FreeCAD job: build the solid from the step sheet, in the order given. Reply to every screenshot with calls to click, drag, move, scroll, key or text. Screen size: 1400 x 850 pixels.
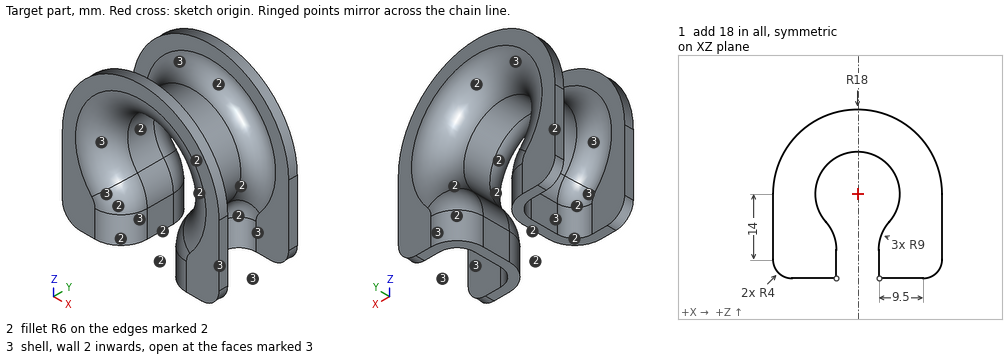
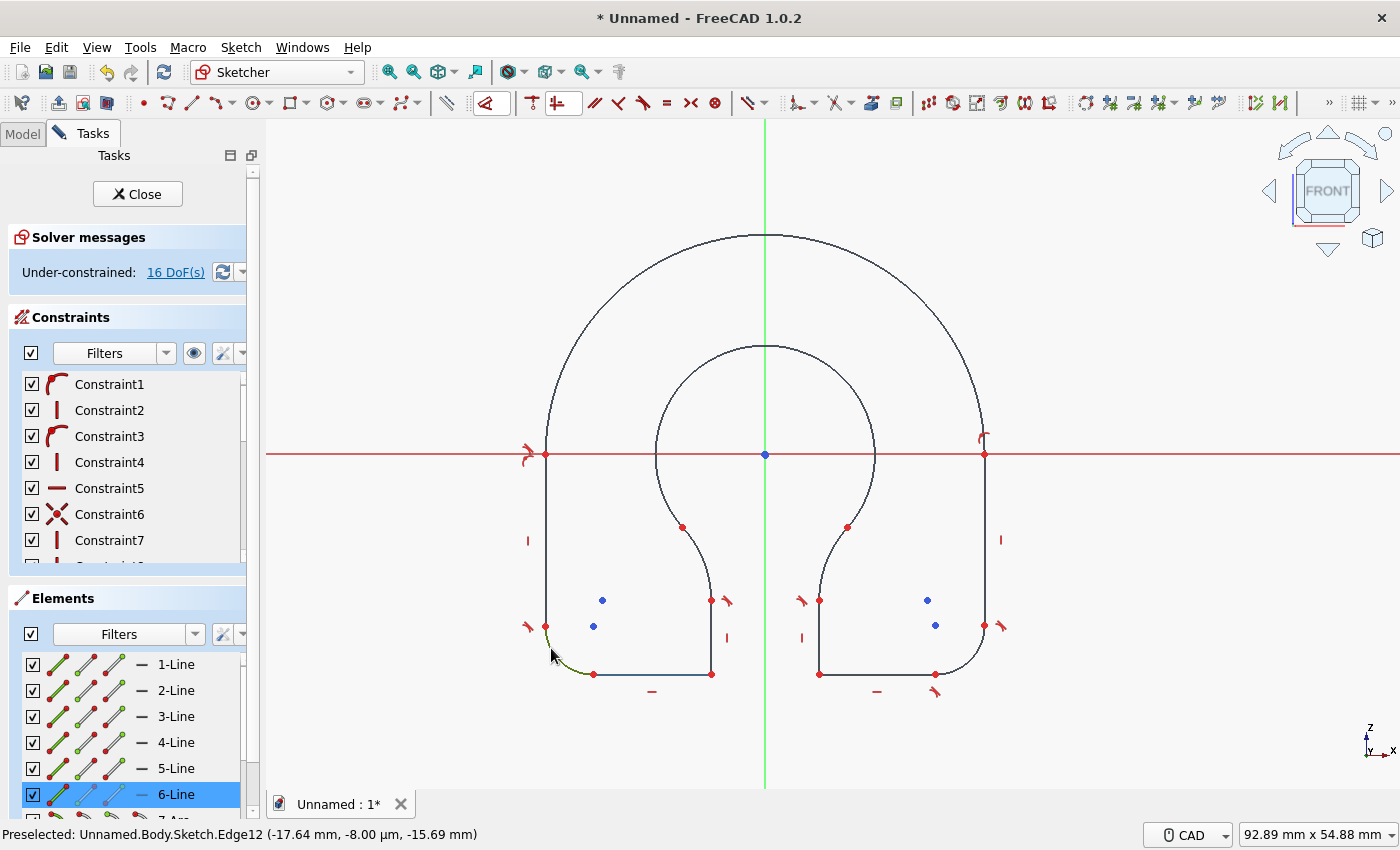
key(t)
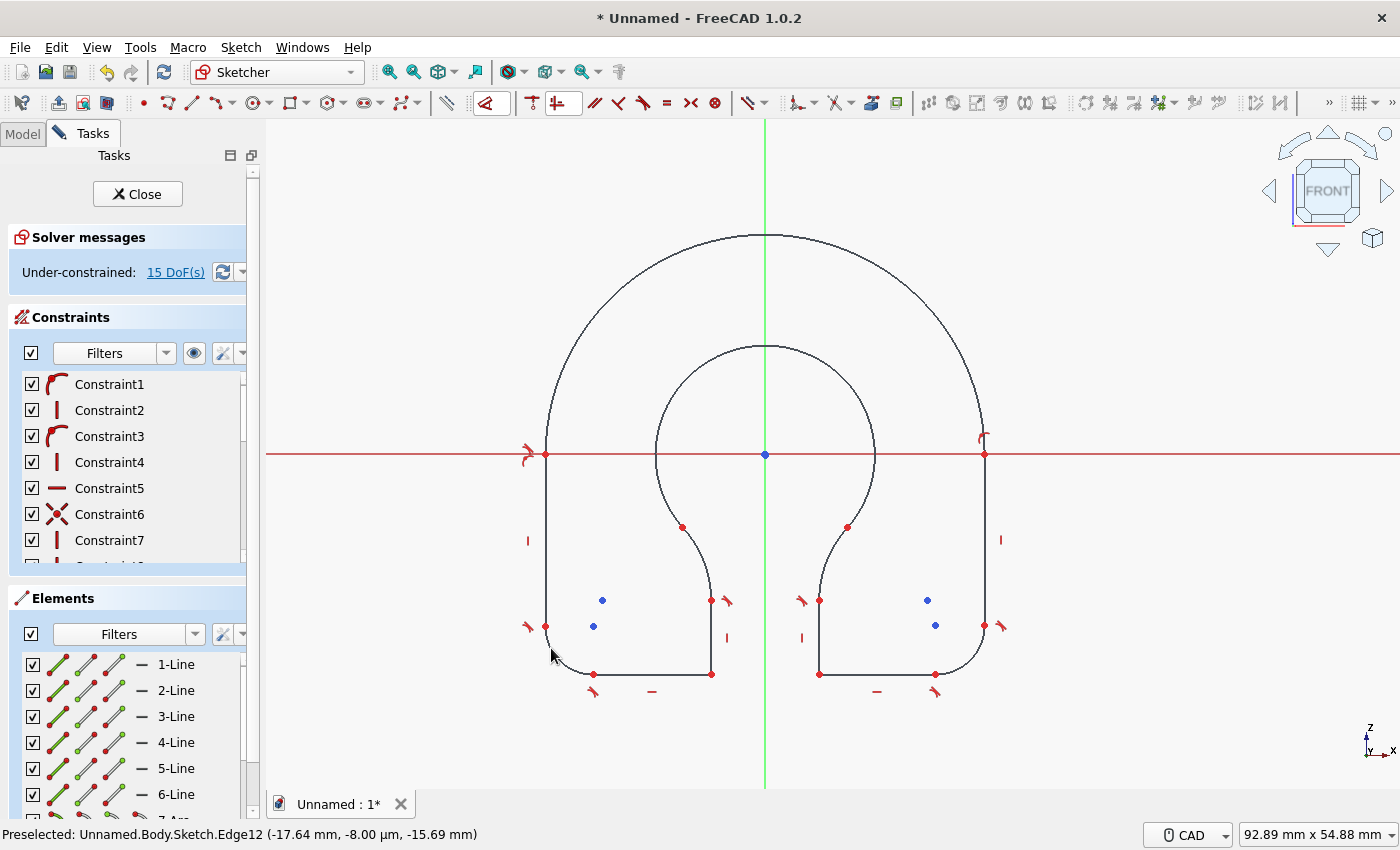
click(833, 547)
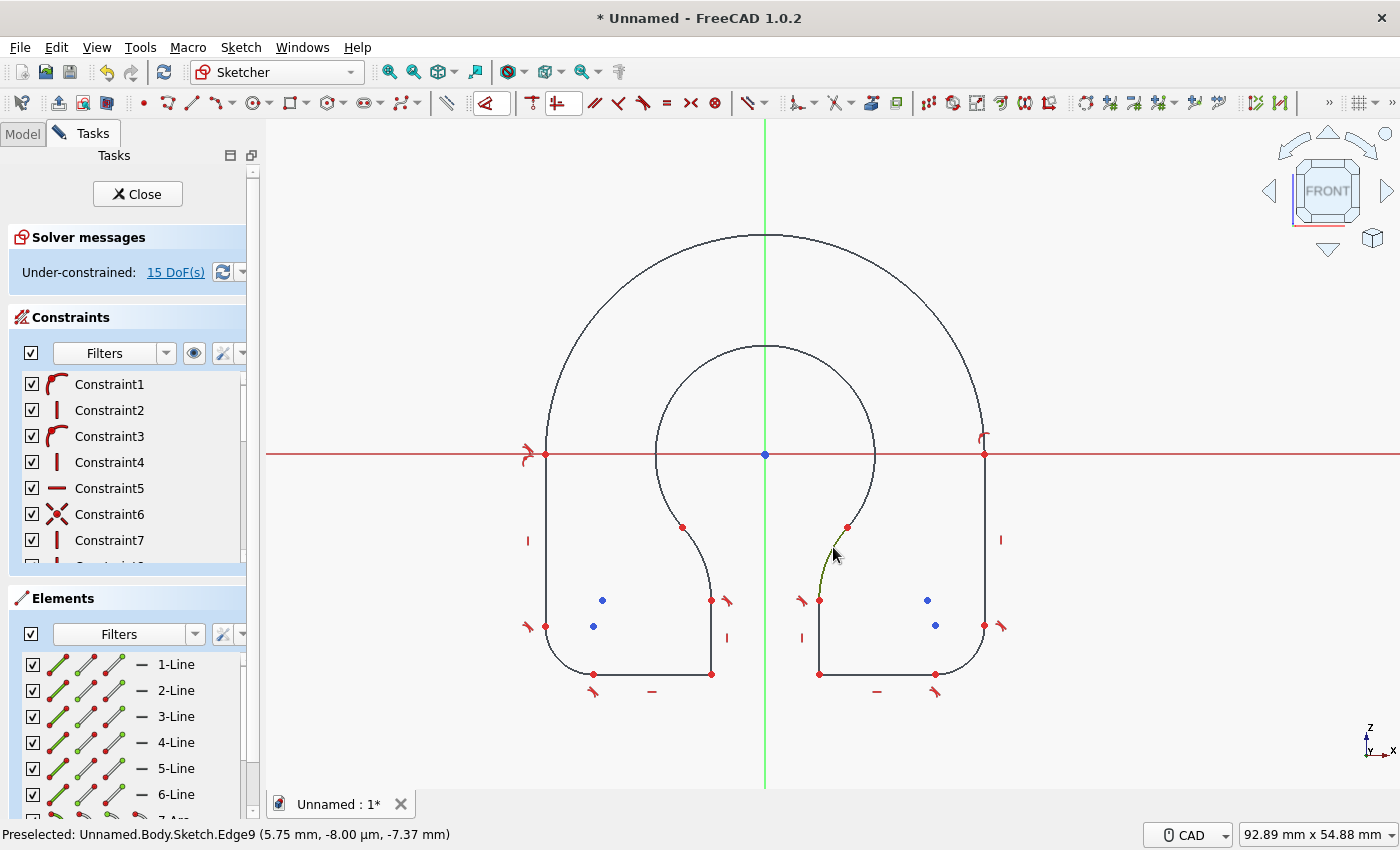
click(852, 389)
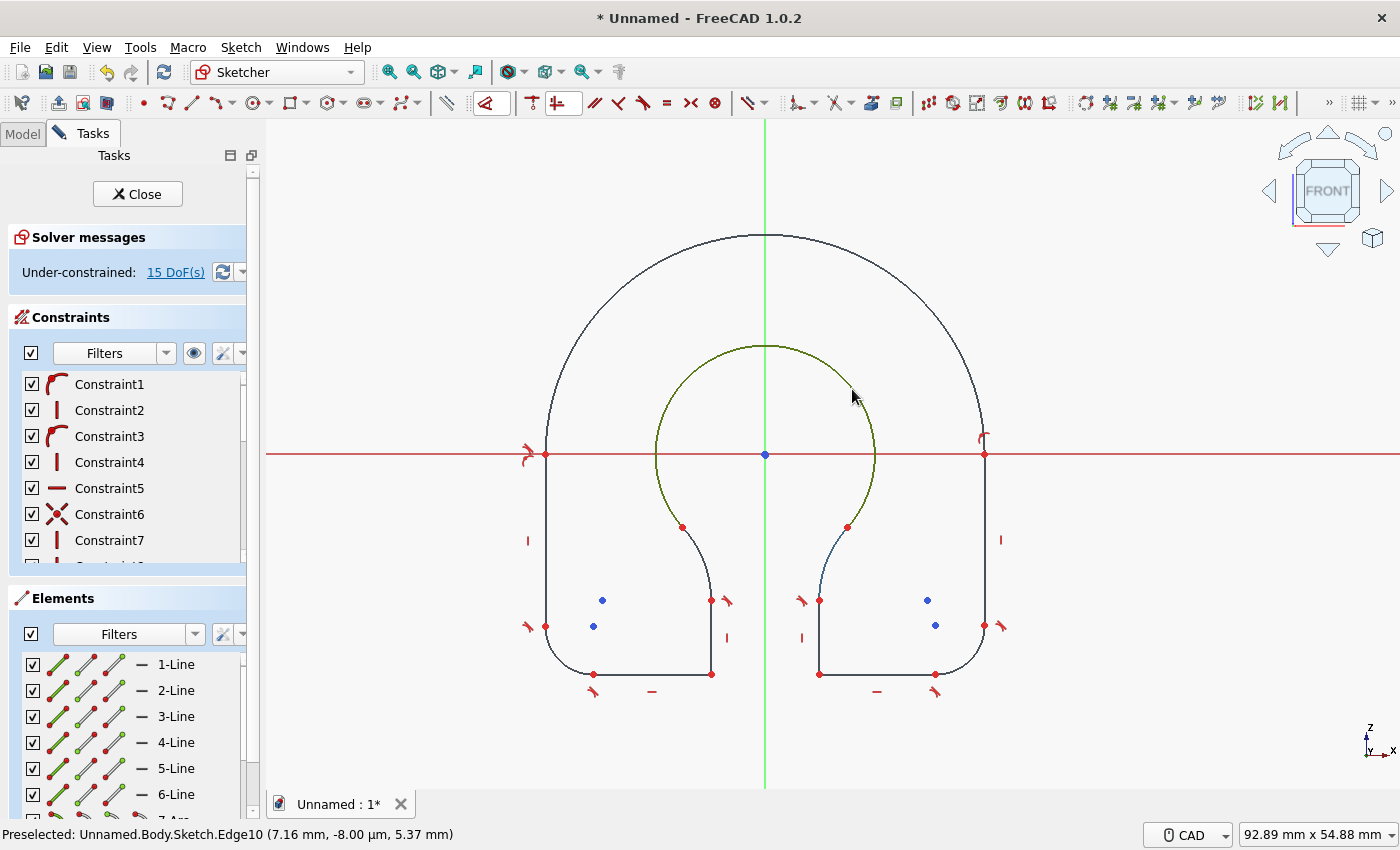
key(t)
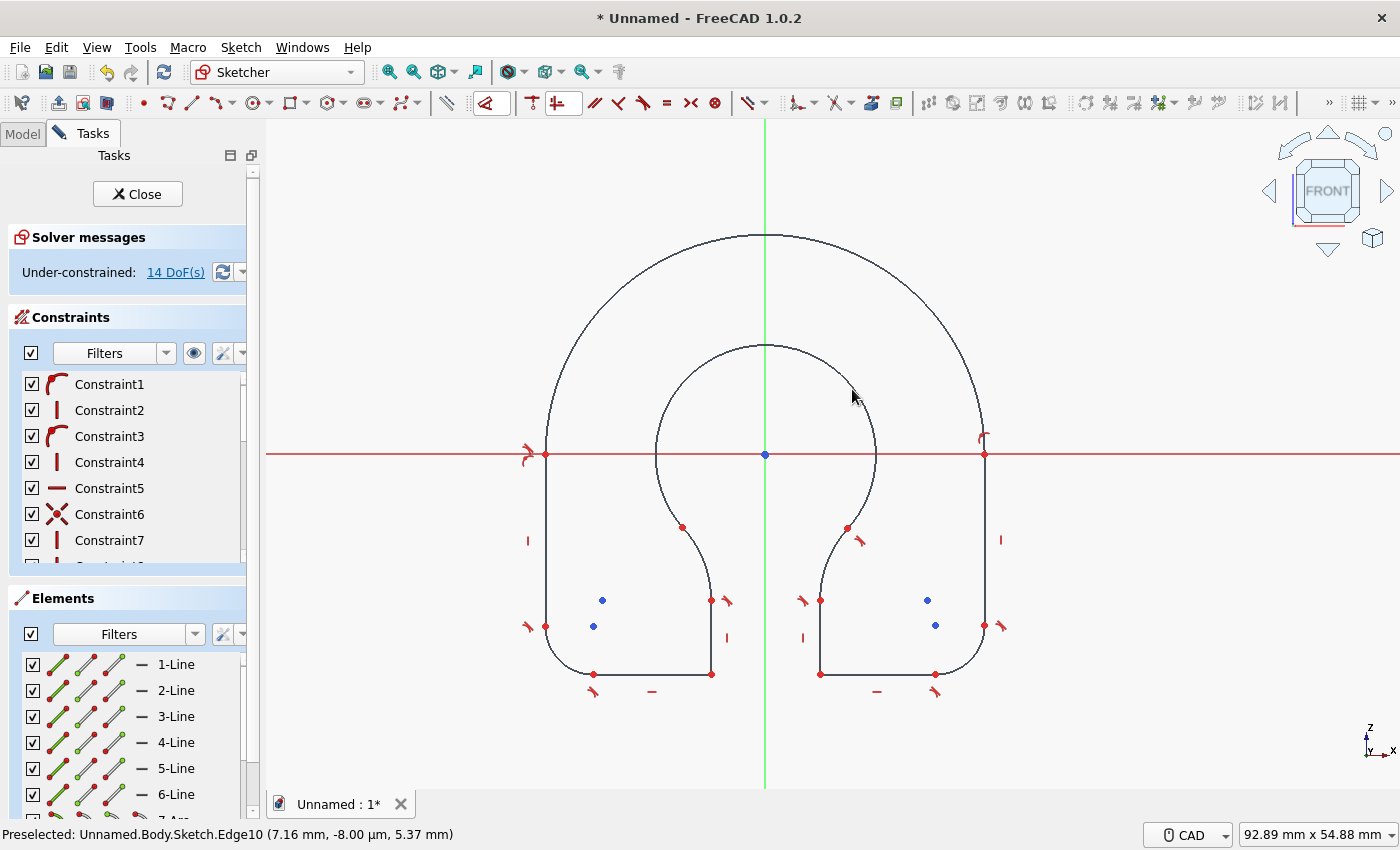
click(854, 389)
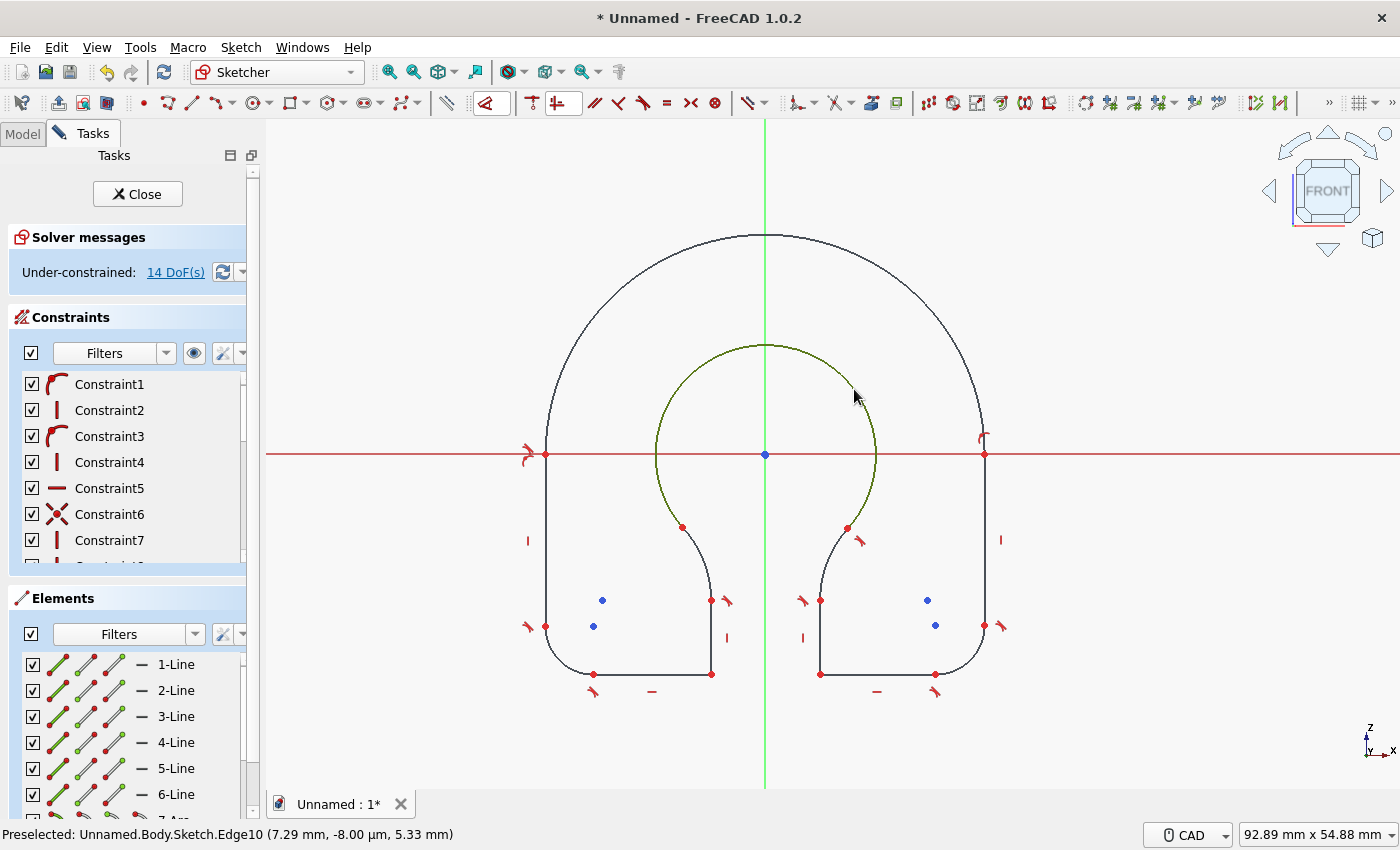
click(708, 577)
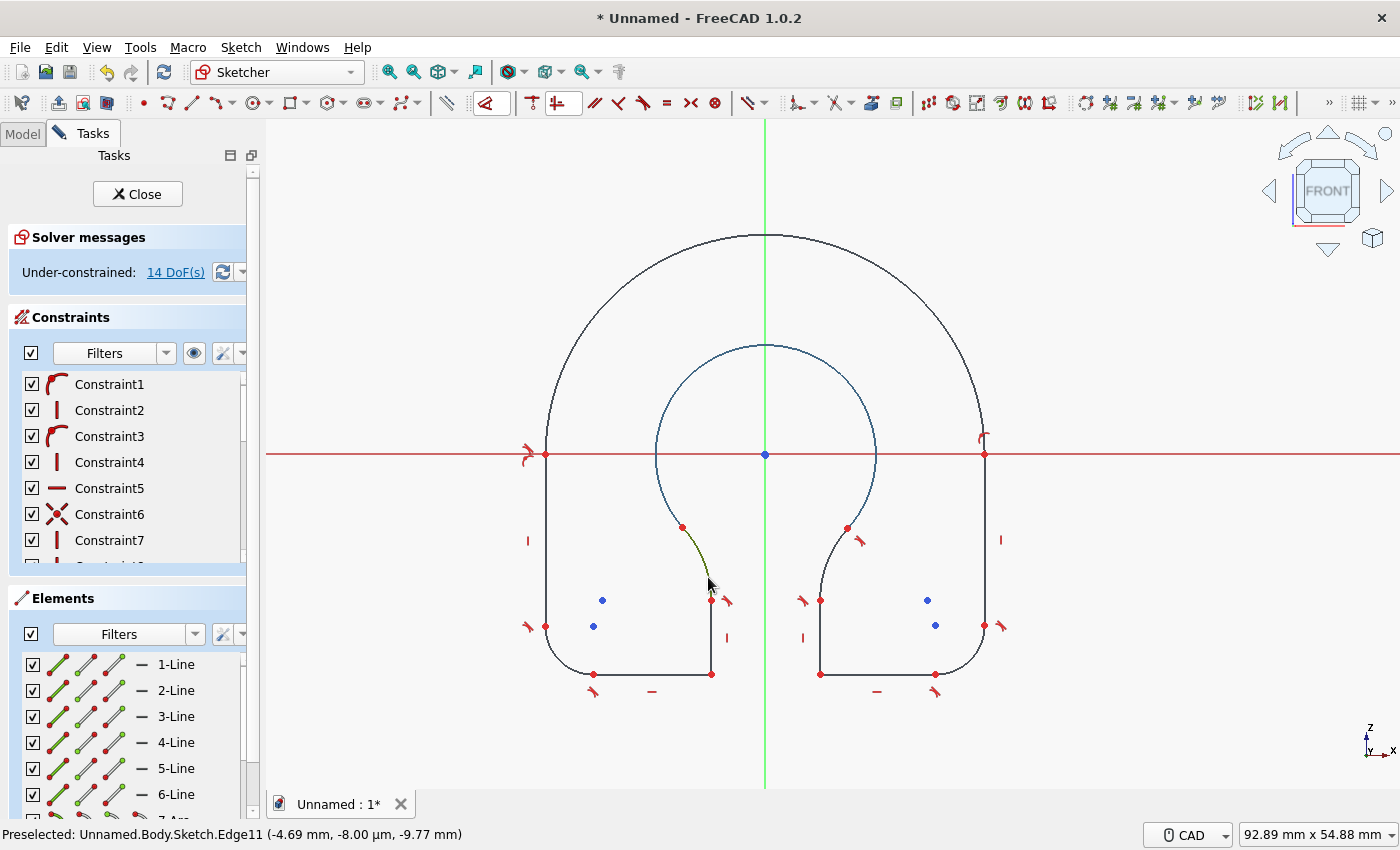
key(t)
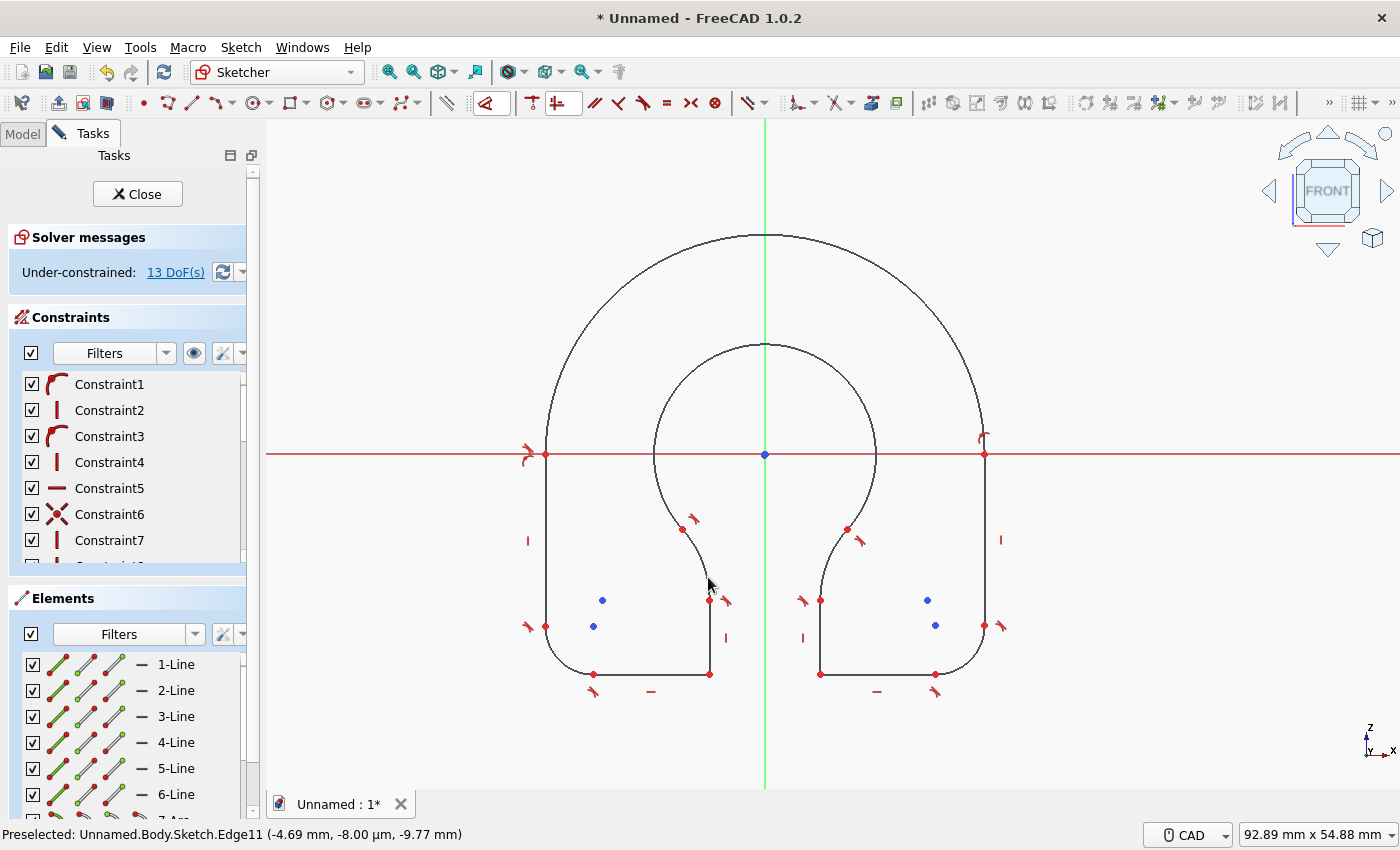
click(894, 277)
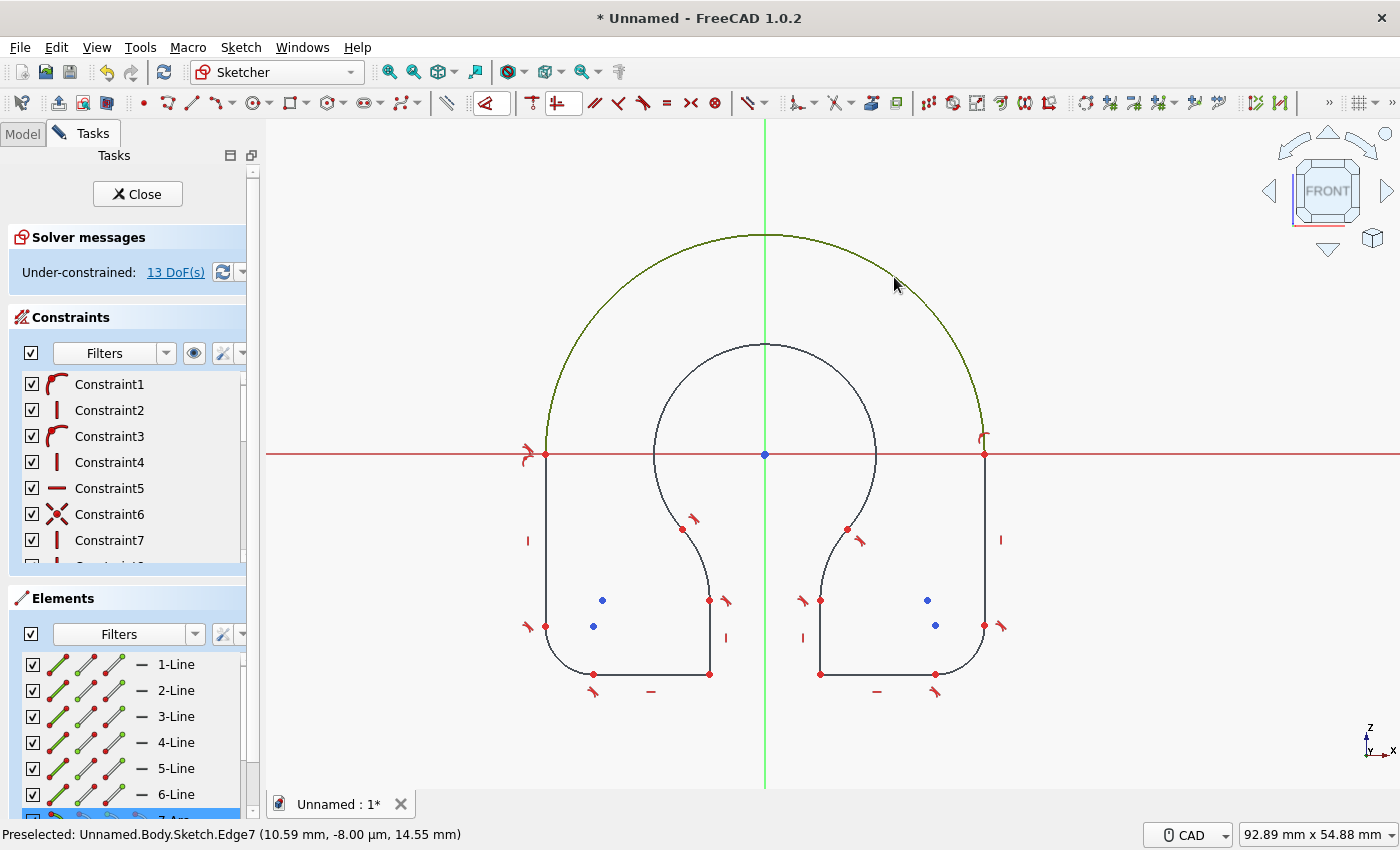
click(853, 388)